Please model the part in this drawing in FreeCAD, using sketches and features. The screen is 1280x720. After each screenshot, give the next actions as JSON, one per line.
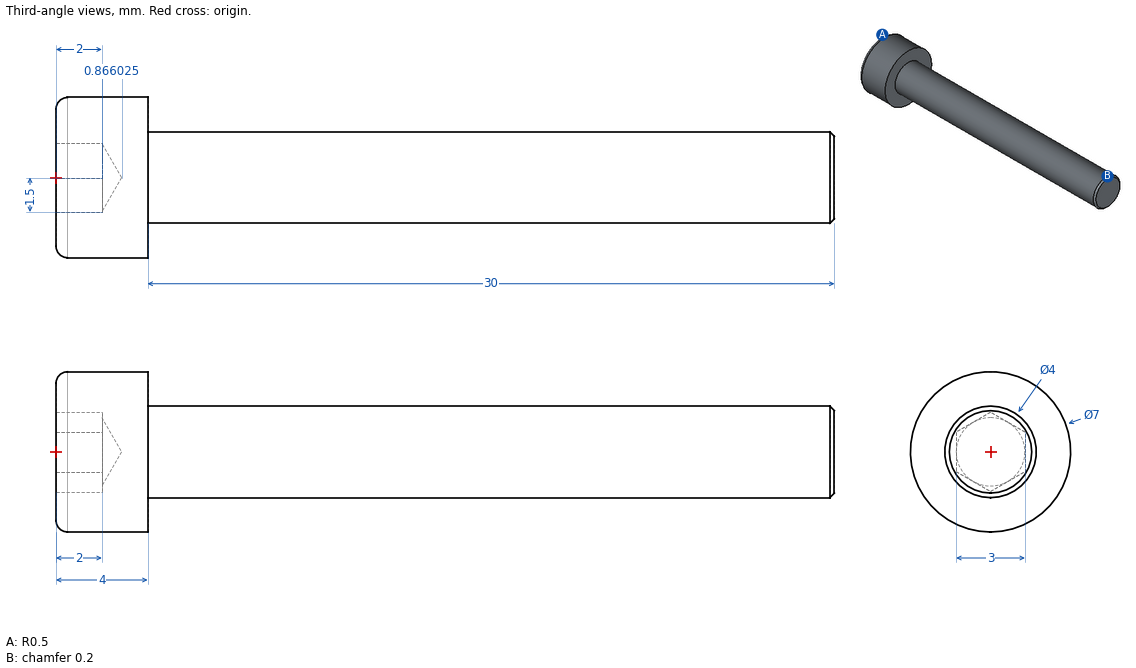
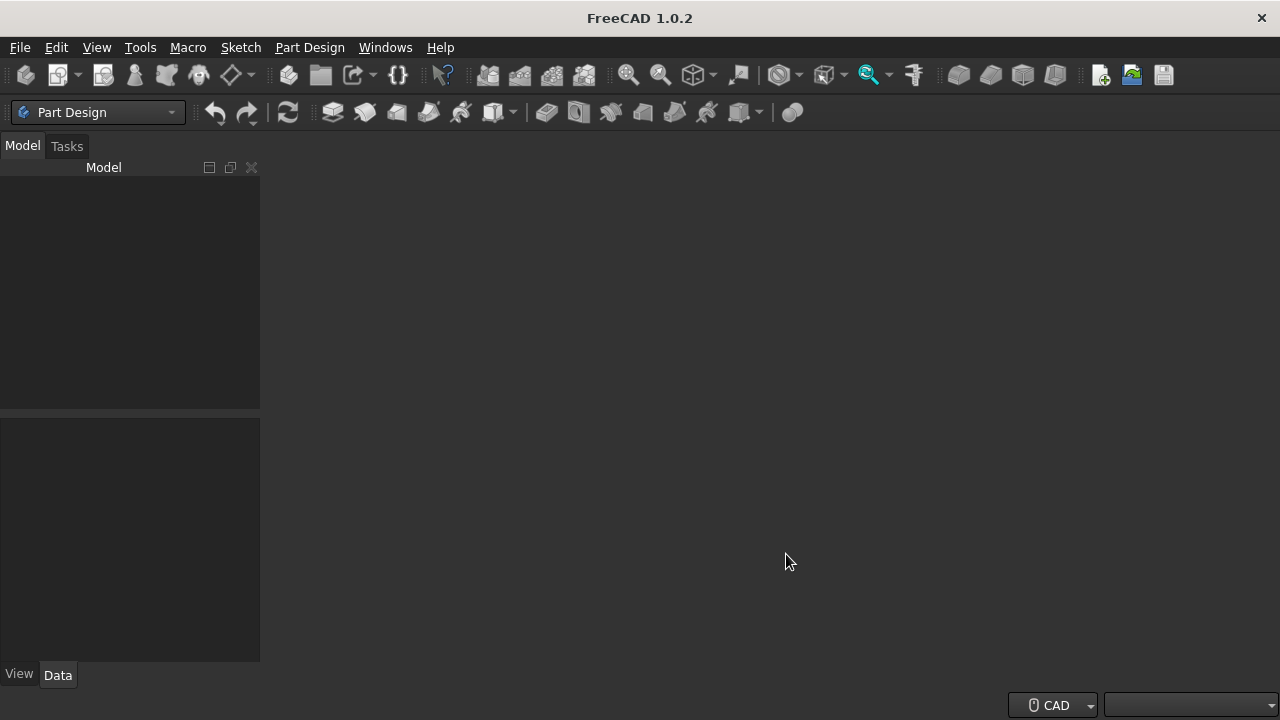
{"action": "left_click", "coordinate": [1100, 76]}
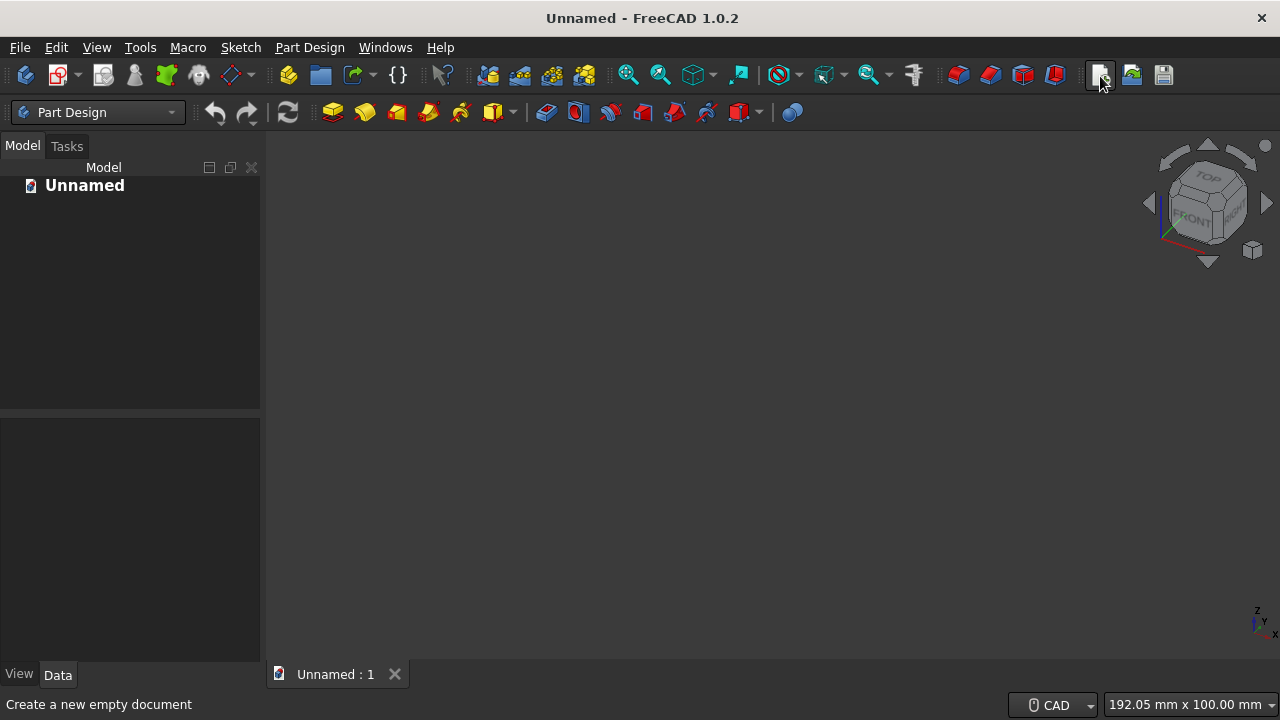
{"action": "left_click", "coordinate": [58, 76]}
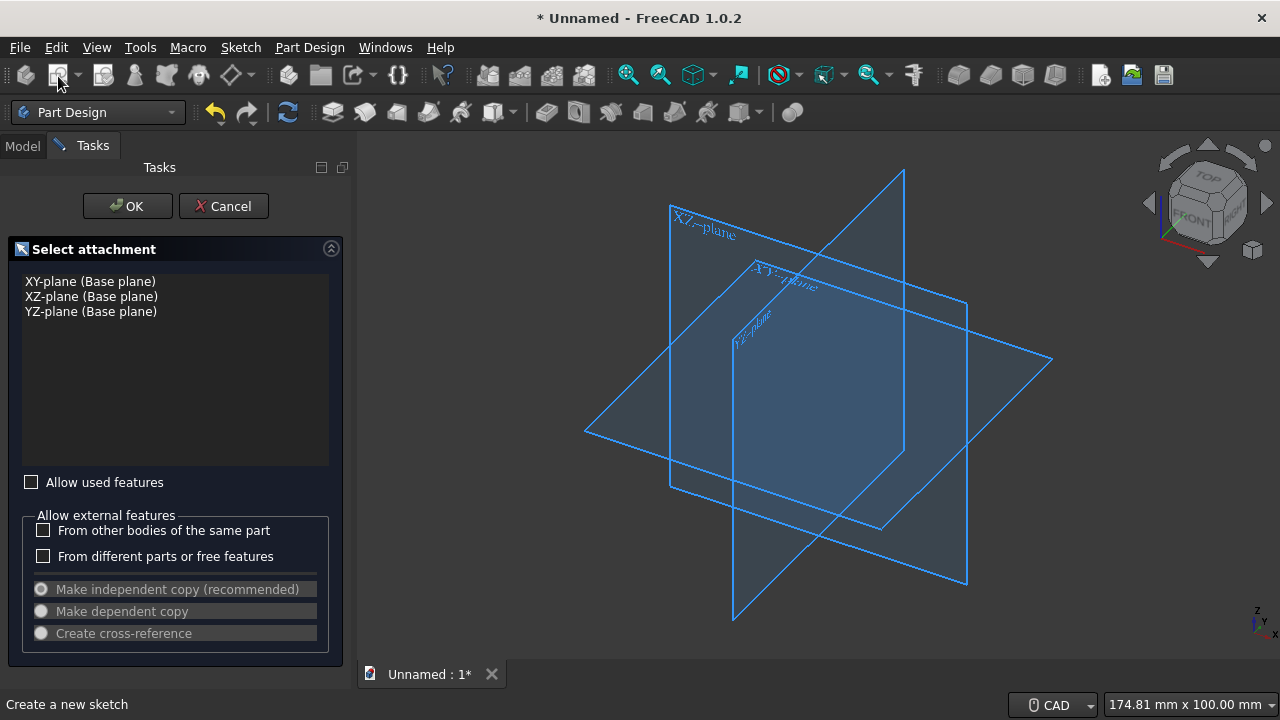
{"action": "left_click", "coordinate": [82, 312]}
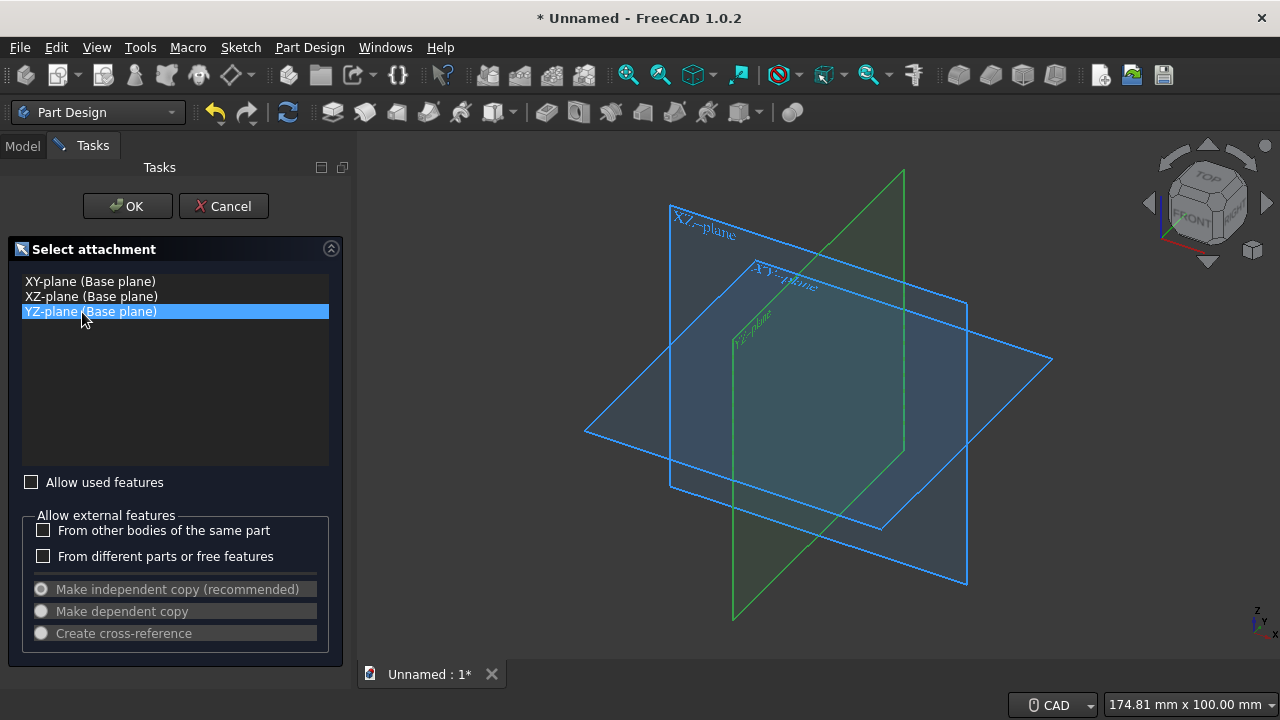
{"action": "left_click", "coordinate": [128, 206]}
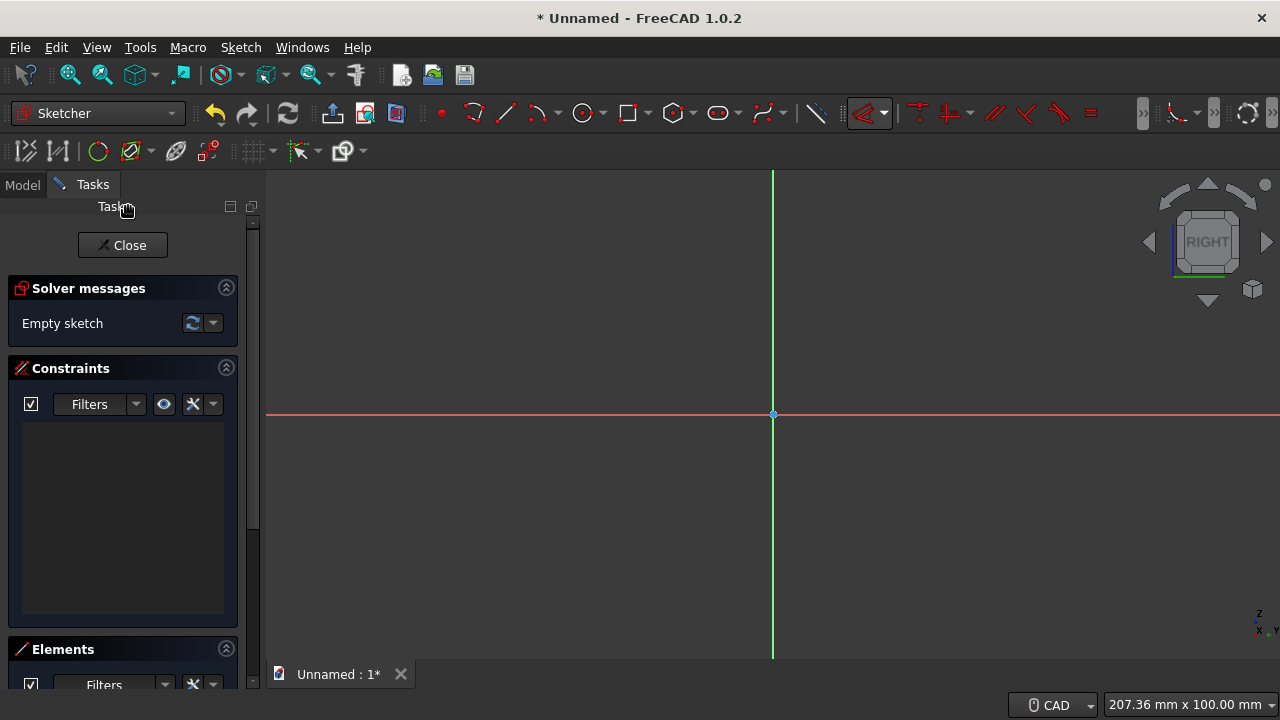
{"action": "scroll", "coordinate": [782, 414], "scroll_direction": "up", "scroll_amount": 11}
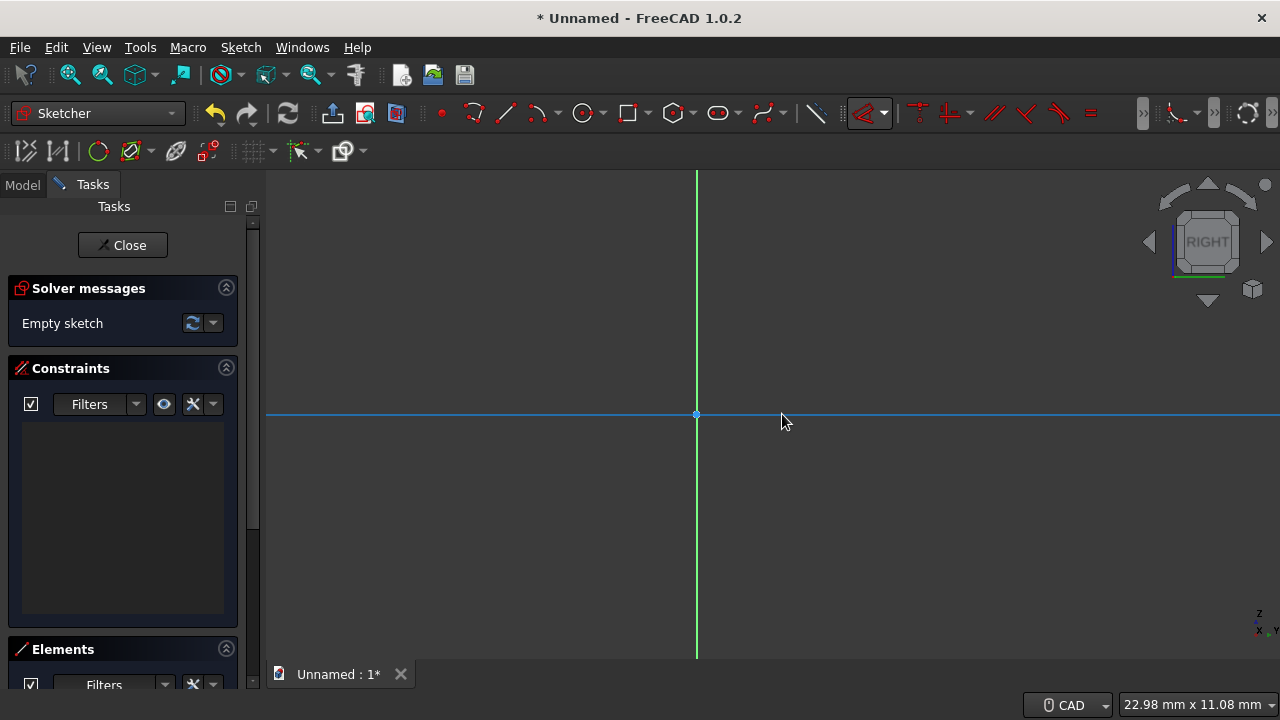
{"action": "left_click", "coordinate": [584, 114]}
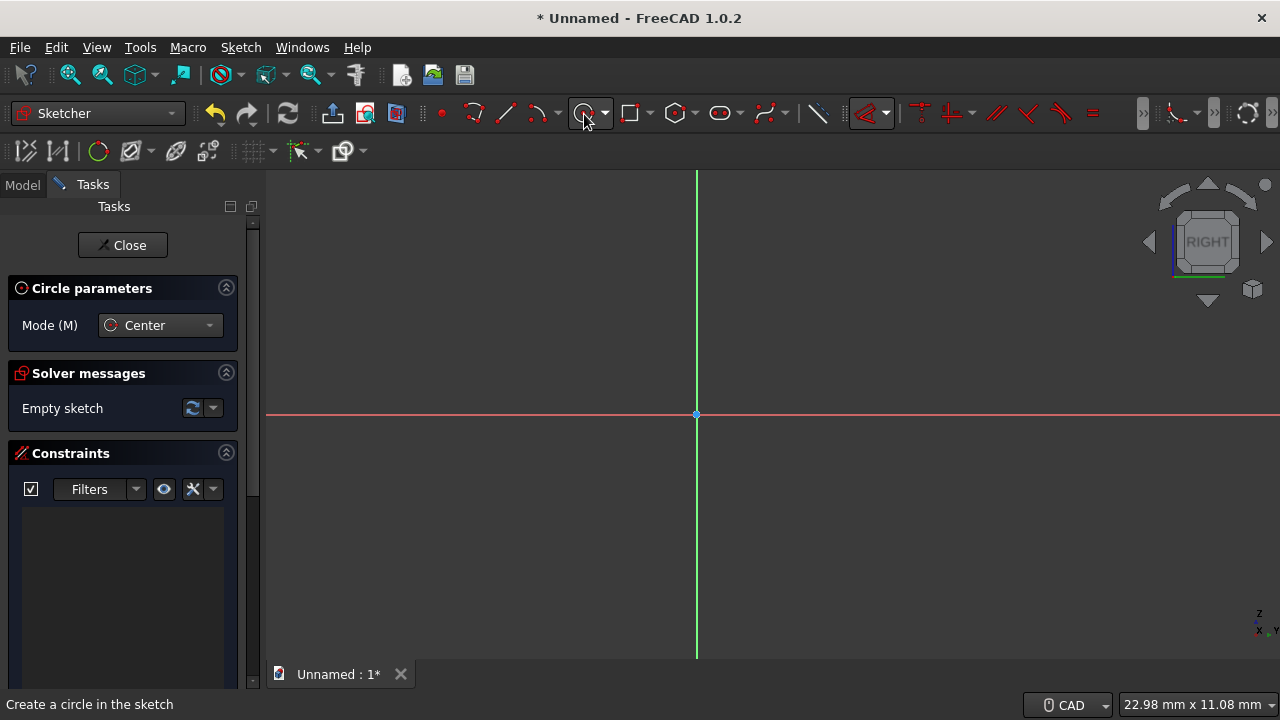
{"action": "left_click", "coordinate": [697, 414]}
{"action": "left_click", "coordinate": [806, 305]}
{"action": "key", "text": "Escape"}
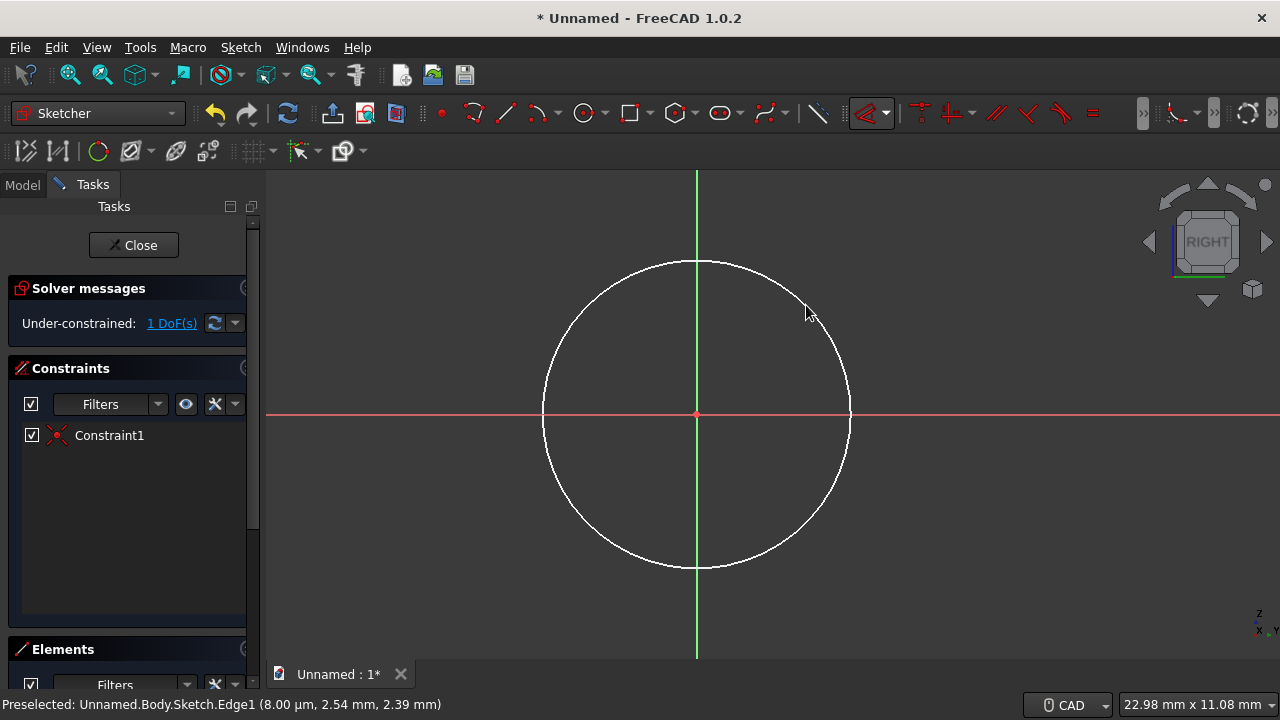
{"action": "left_click", "coordinate": [866, 114]}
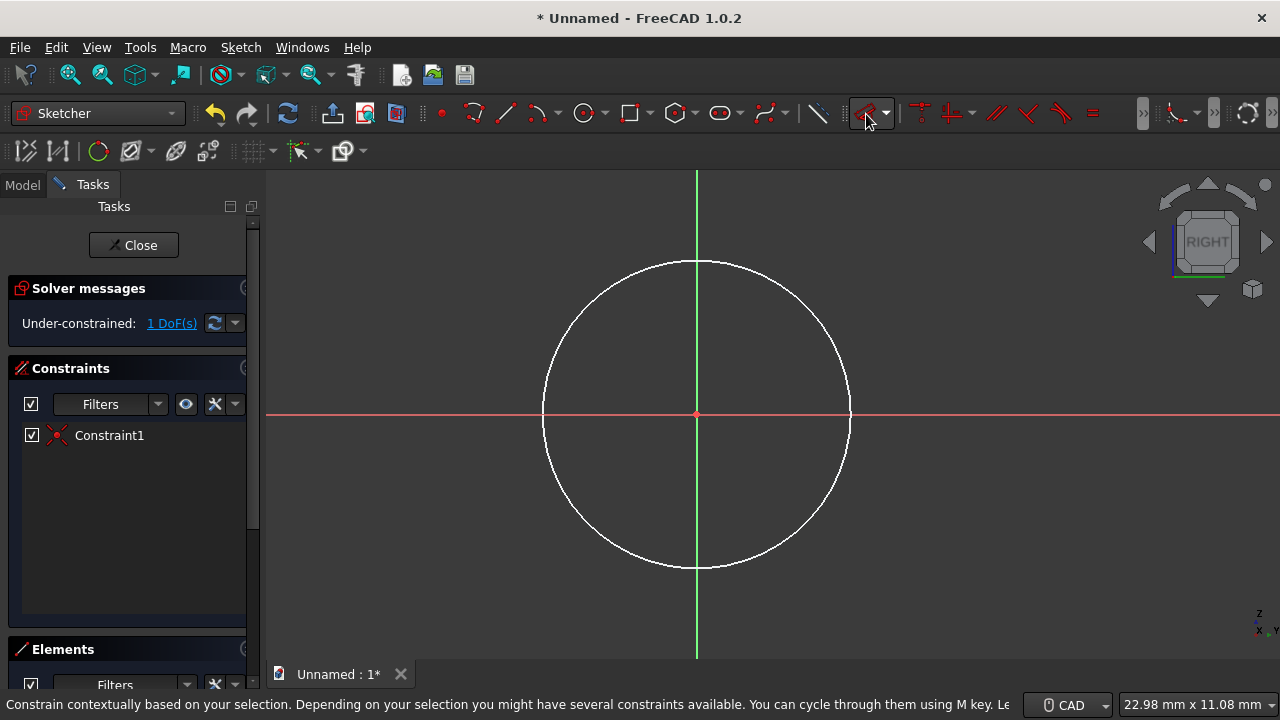
{"action": "left_click", "coordinate": [805, 305]}
{"action": "left_click", "coordinate": [828, 282]}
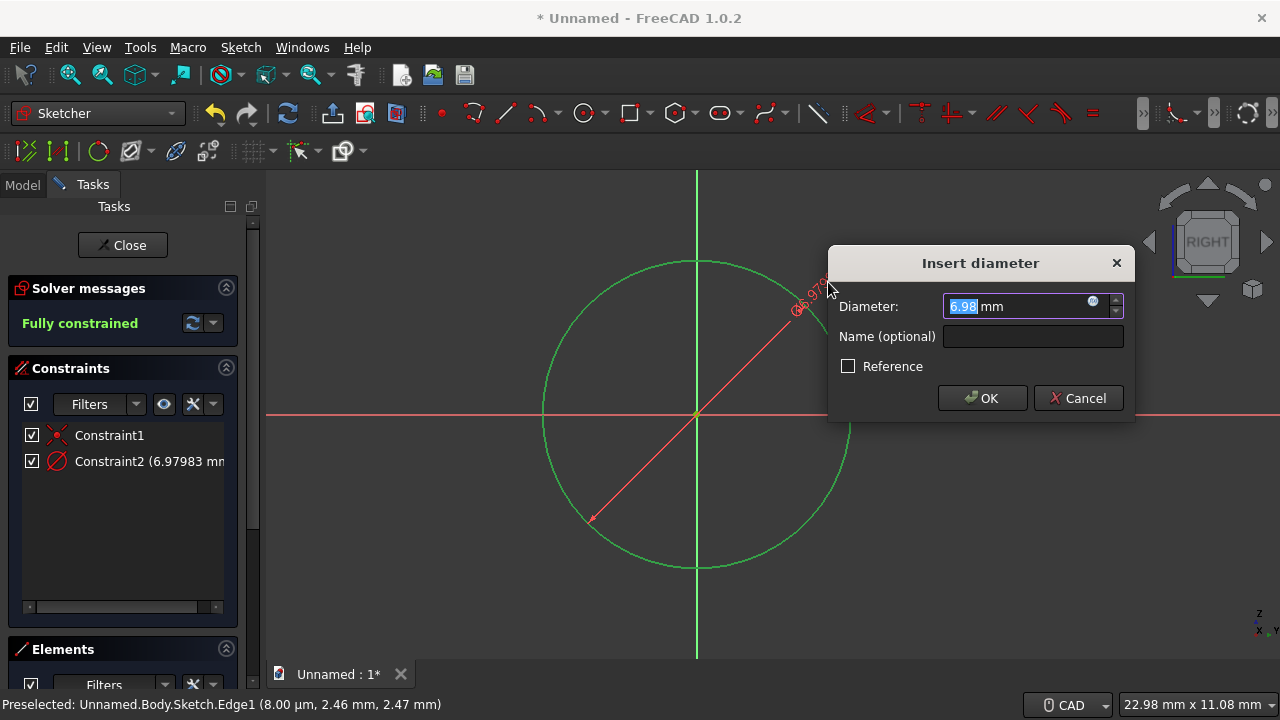
{"action": "type", "text": "7"}
{"action": "key", "text": "Return"}
{"action": "key", "text": "Escape"}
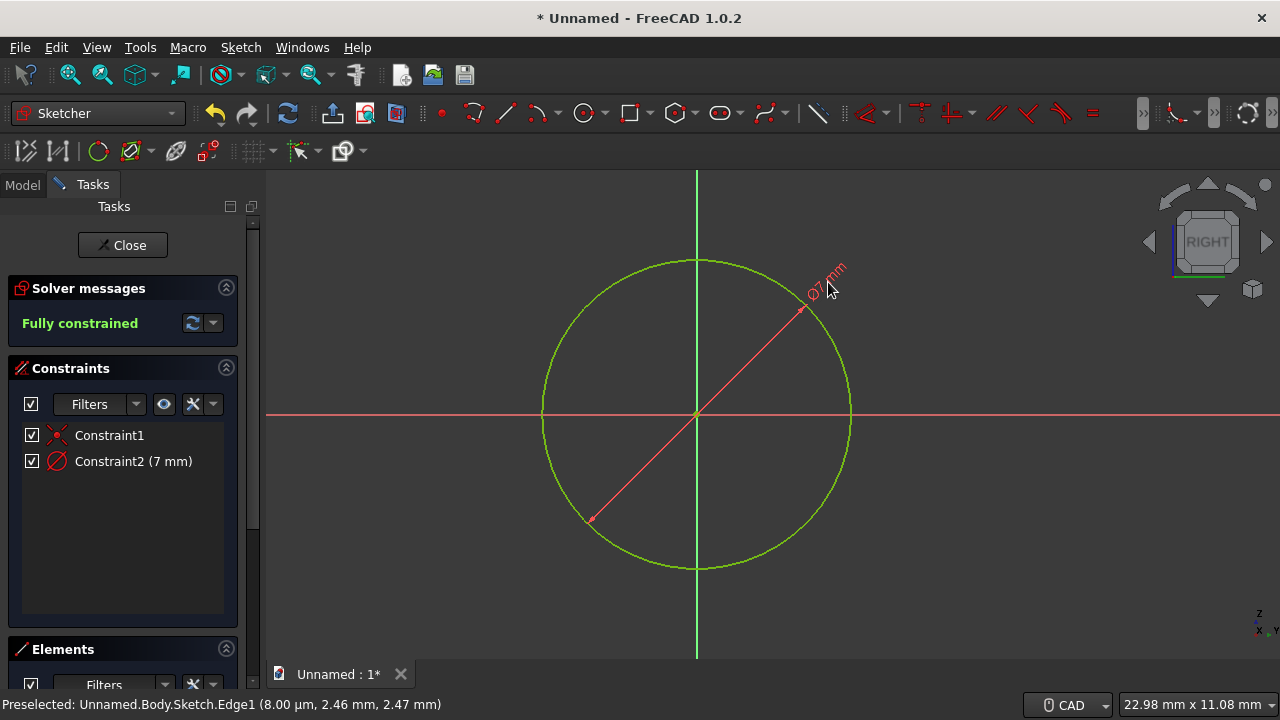
{"action": "left_click", "coordinate": [123, 245]}